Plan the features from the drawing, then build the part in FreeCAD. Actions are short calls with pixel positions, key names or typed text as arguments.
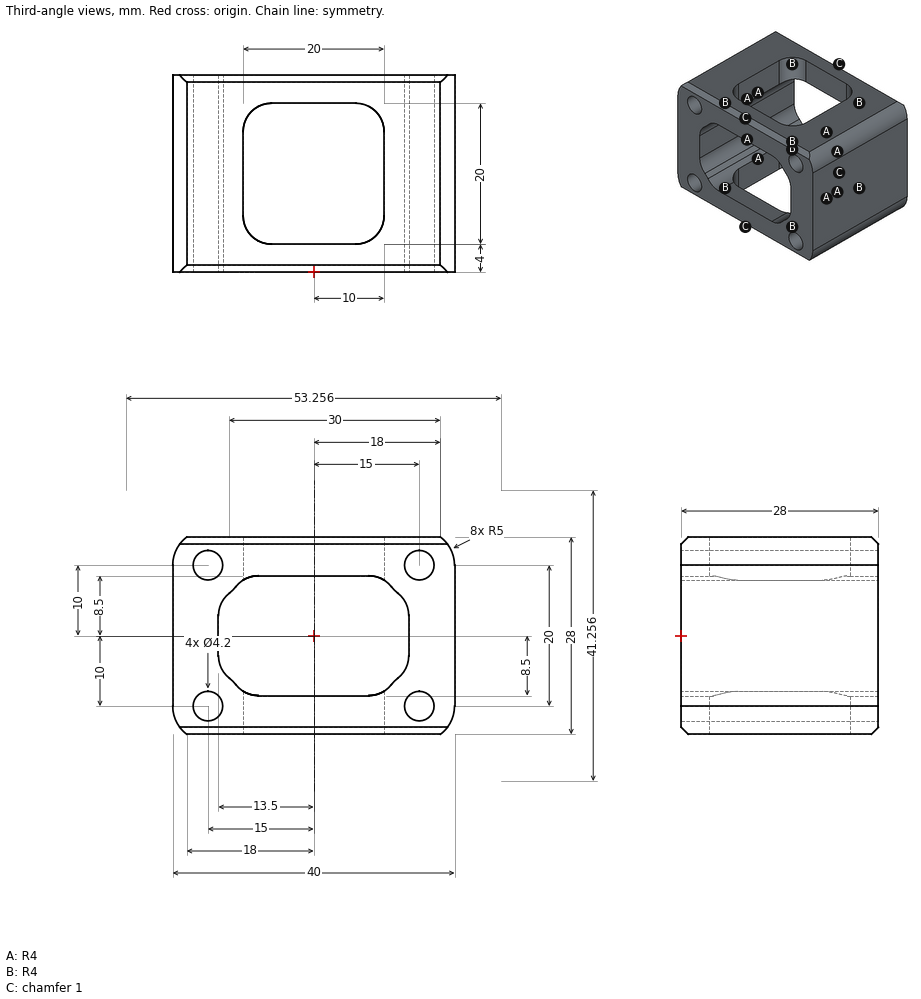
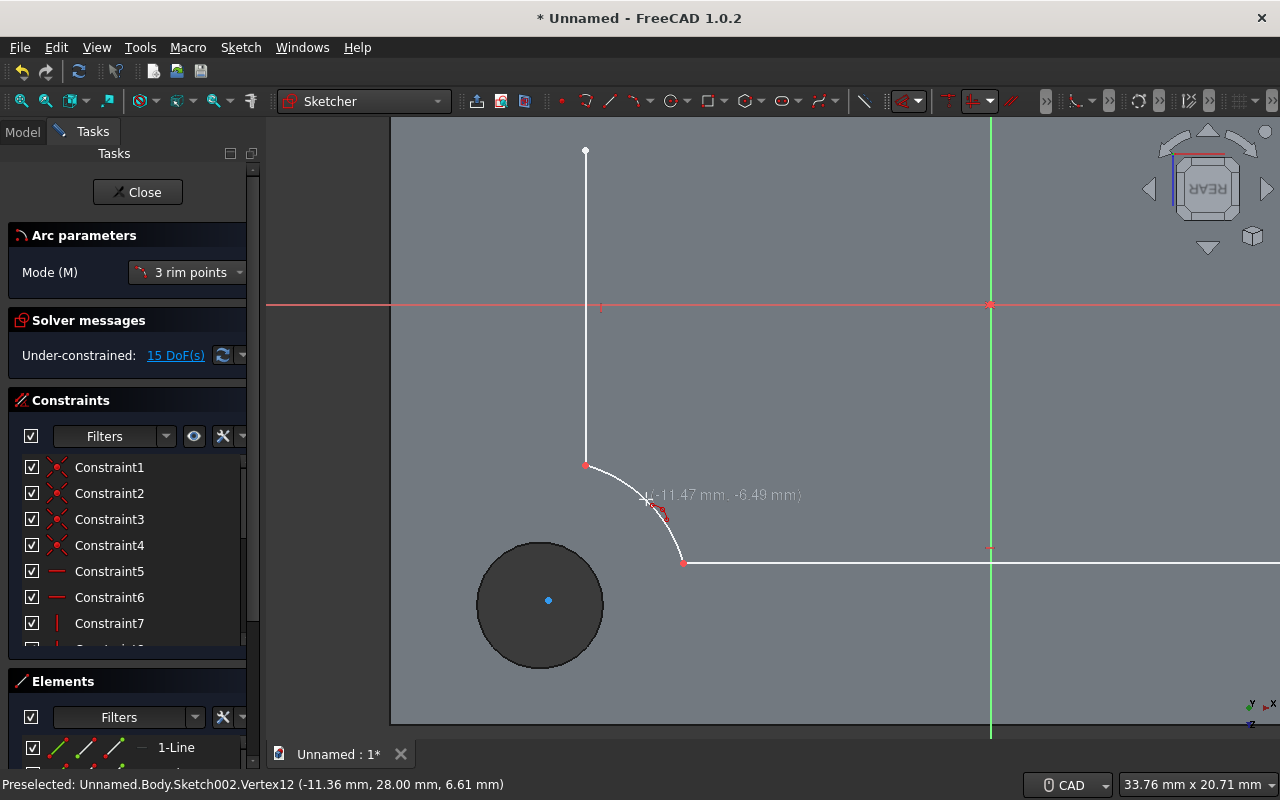
scroll(581, 481, down, 6)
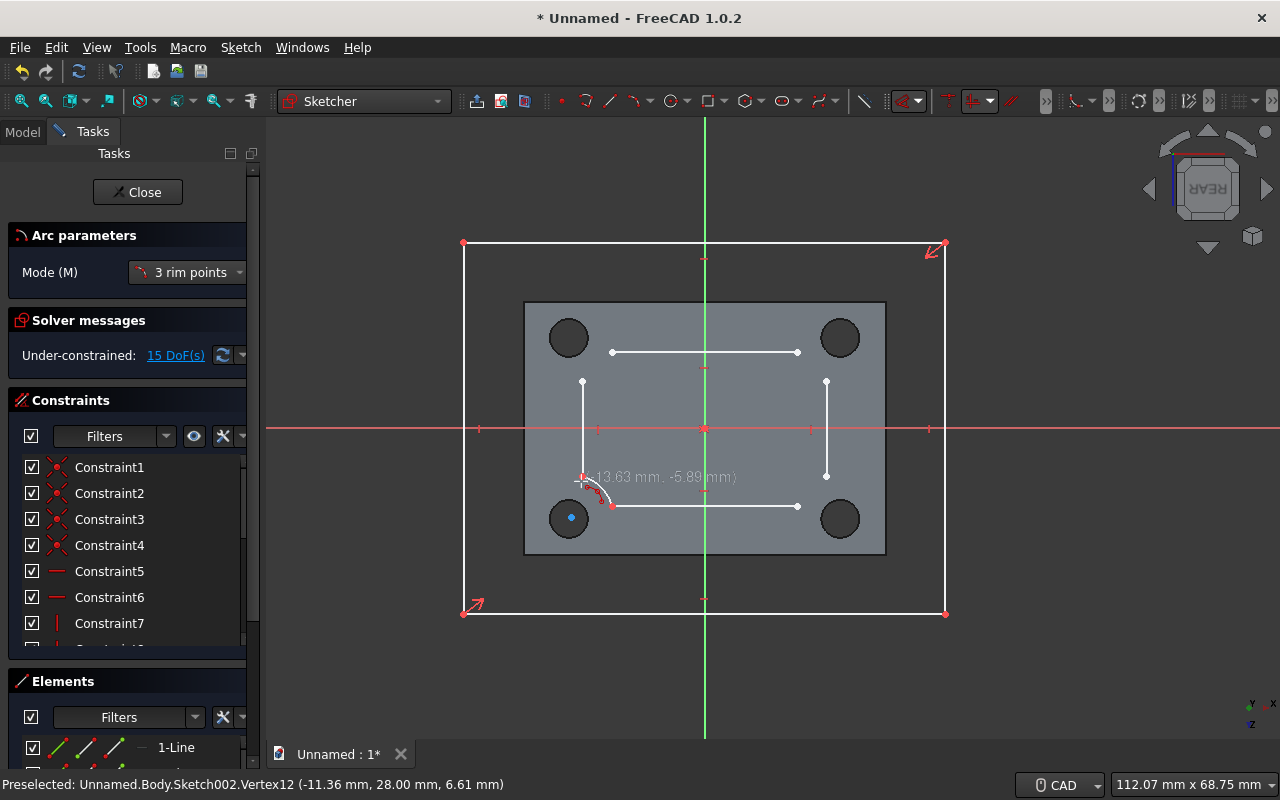
click(797, 506)
click(827, 477)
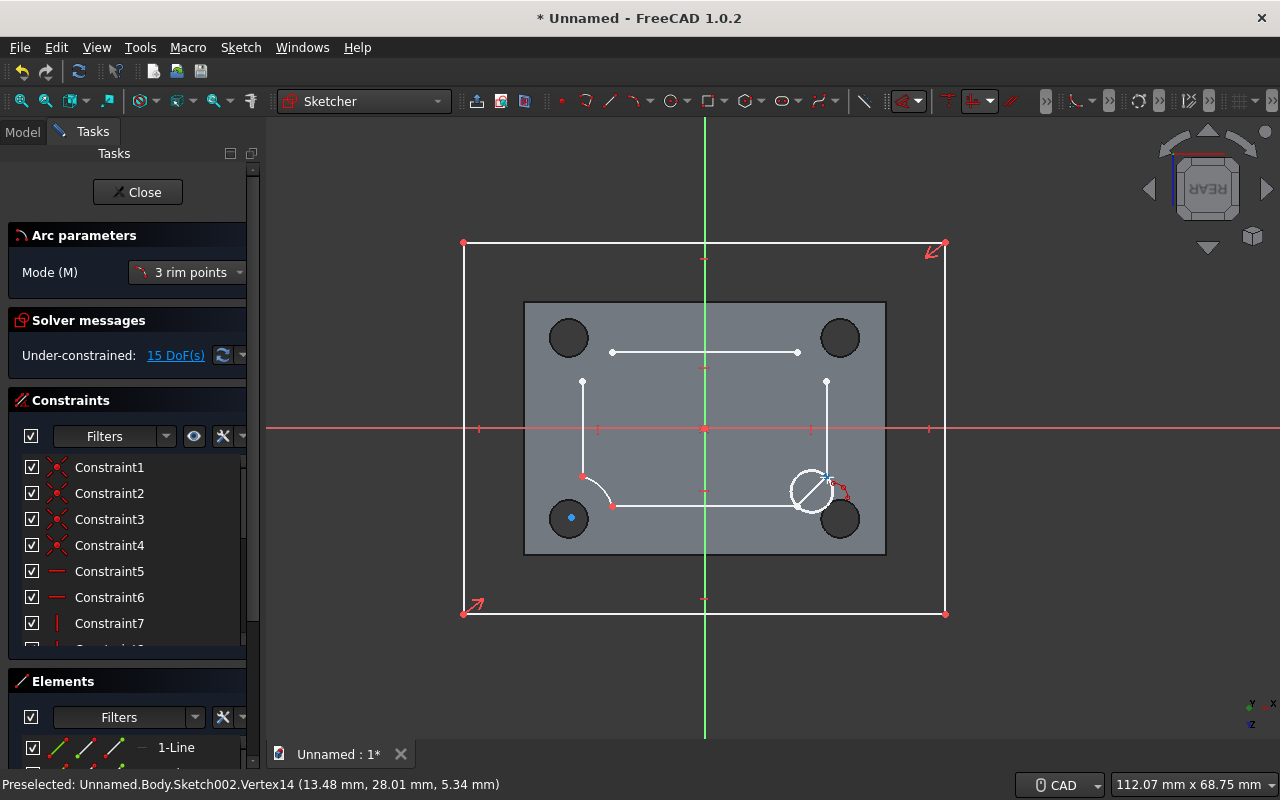
scroll(808, 487, up, 6)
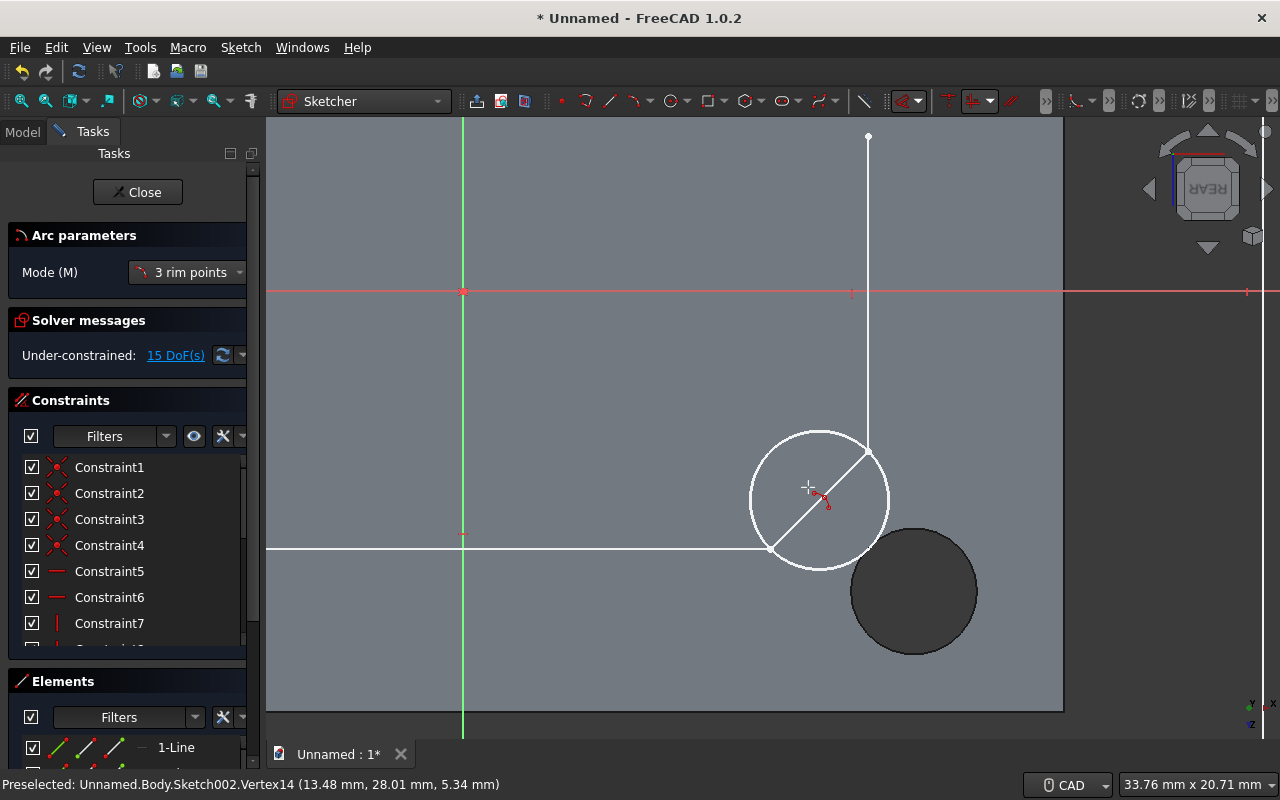
click(808, 485)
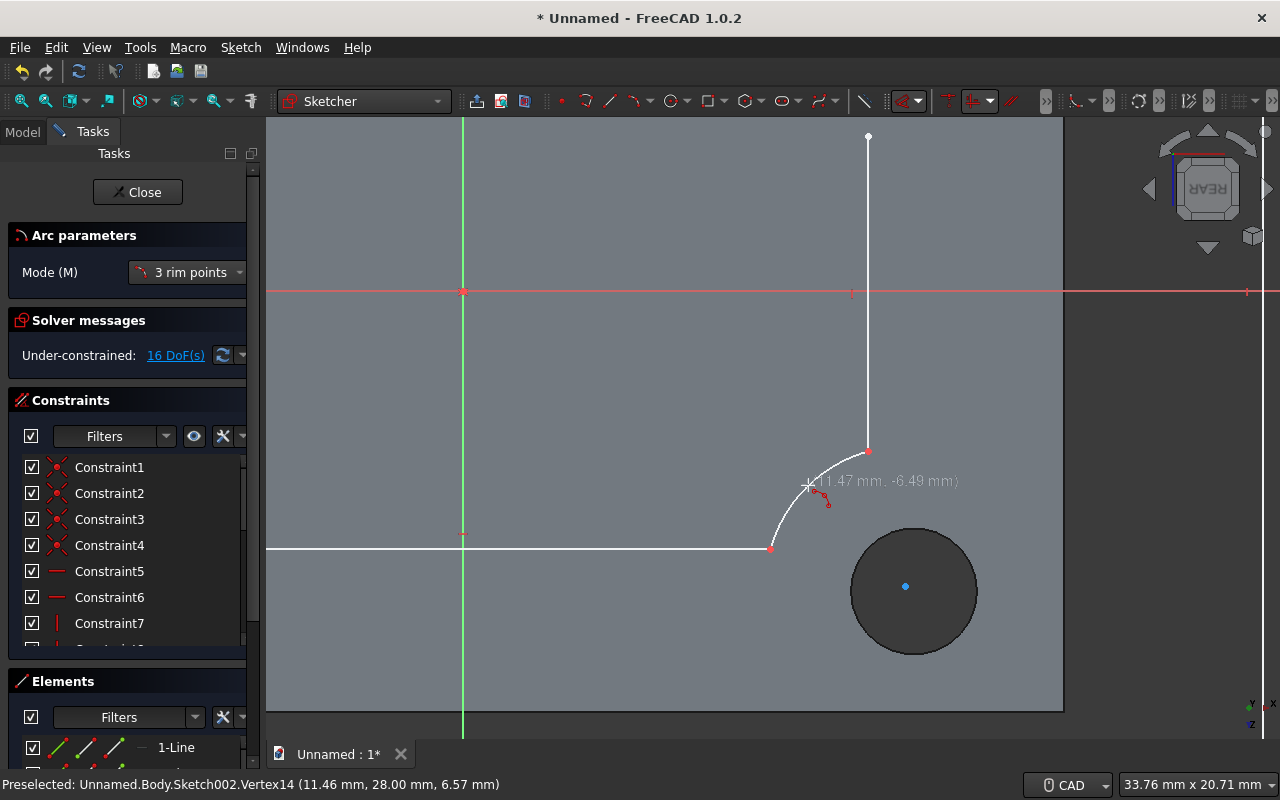
scroll(808, 487, down, 6)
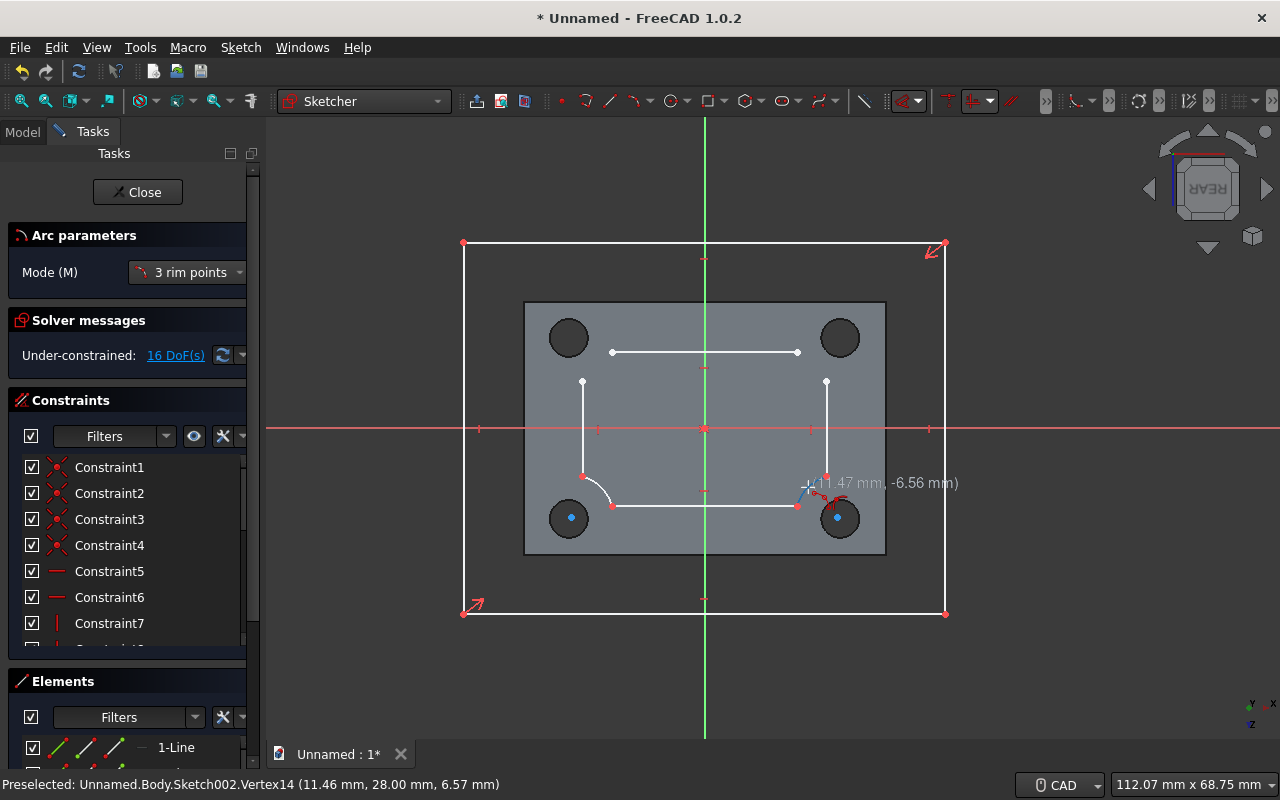
click(827, 382)
click(797, 352)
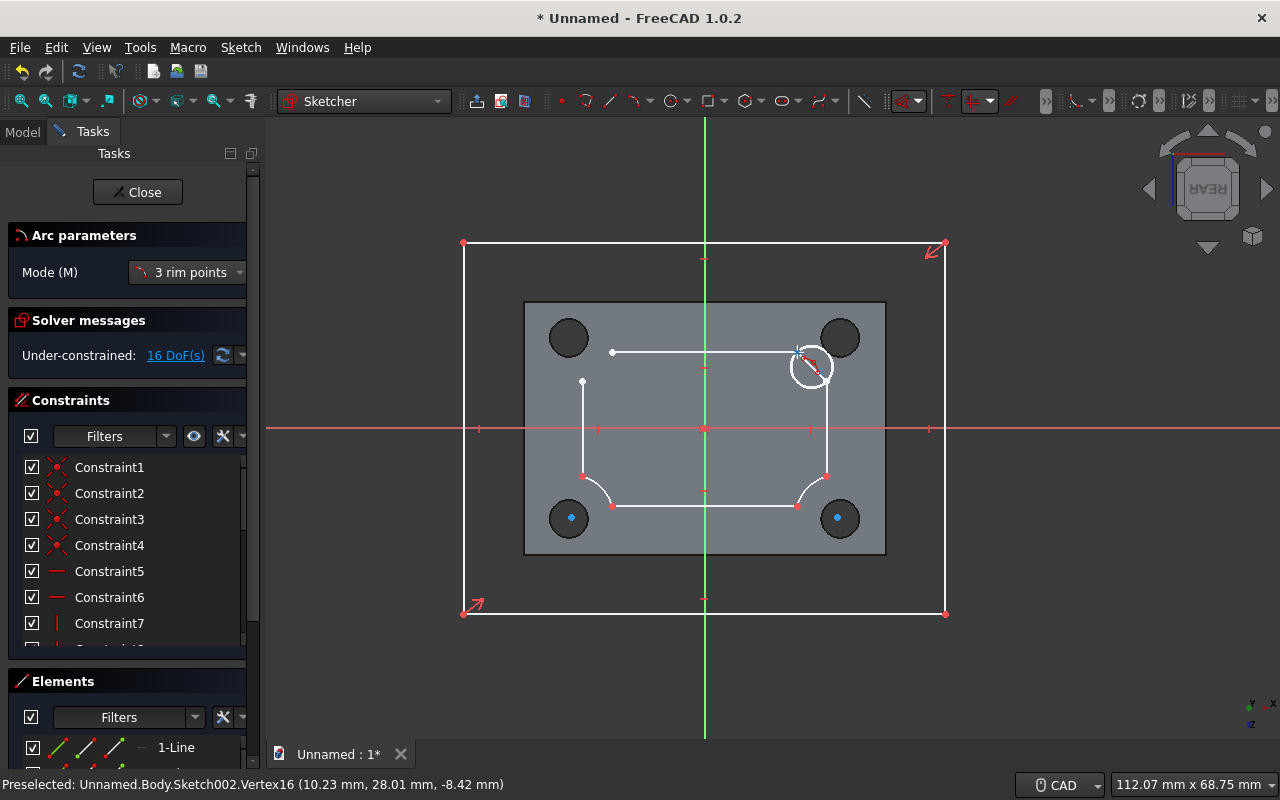
scroll(808, 370, up, 6)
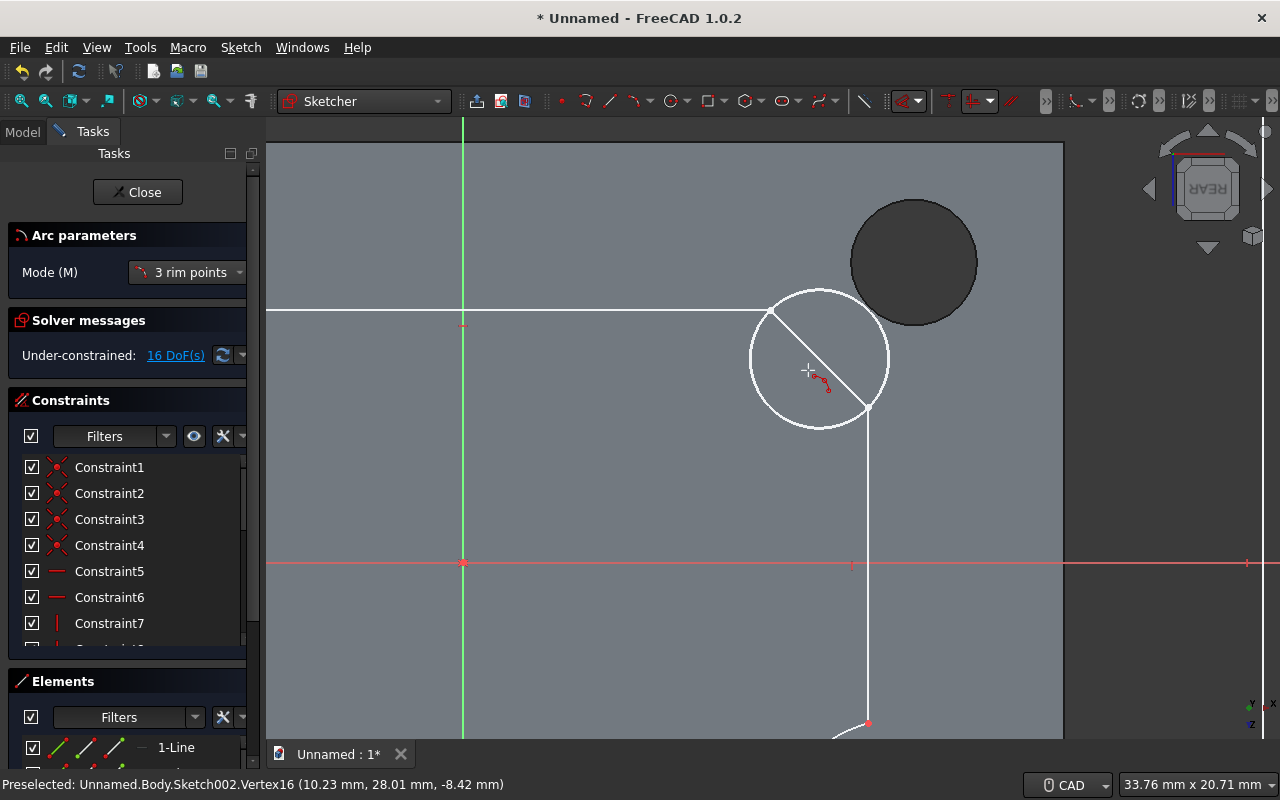
click(808, 369)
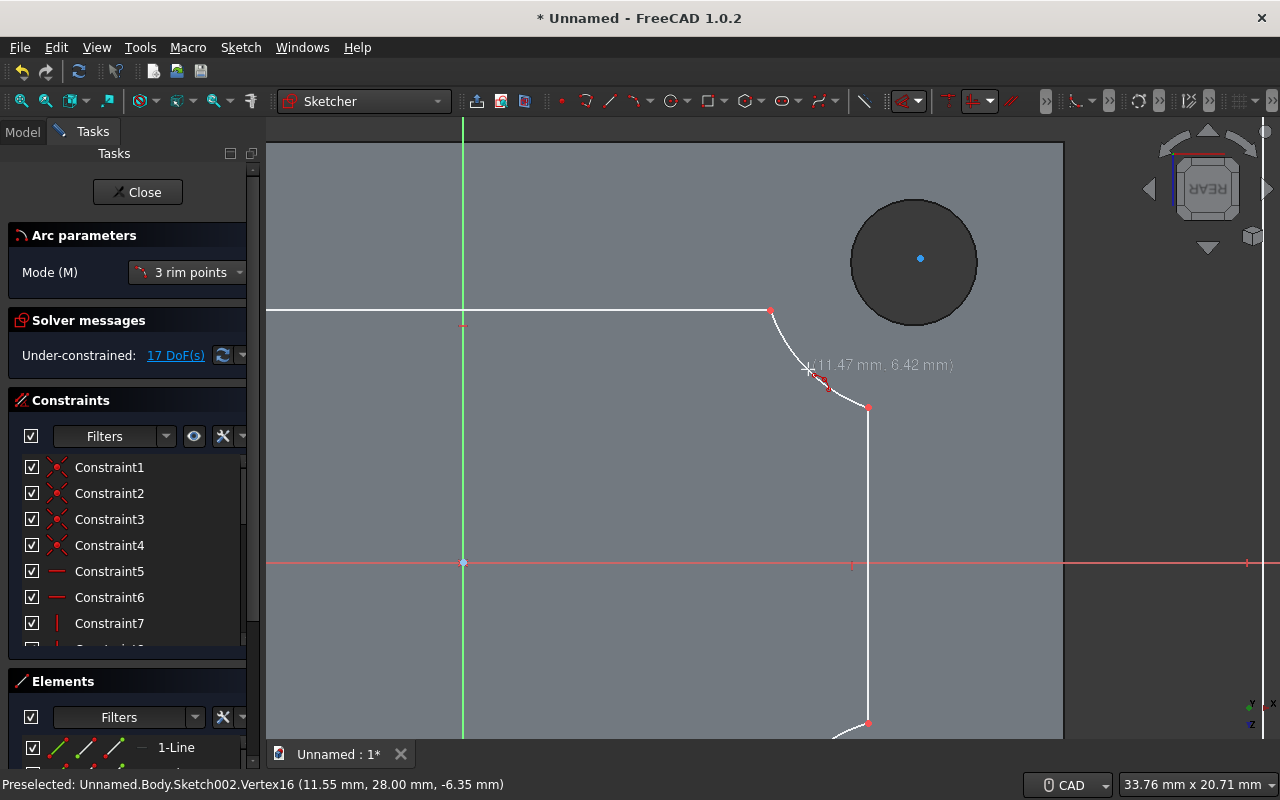
scroll(808, 370, down, 6)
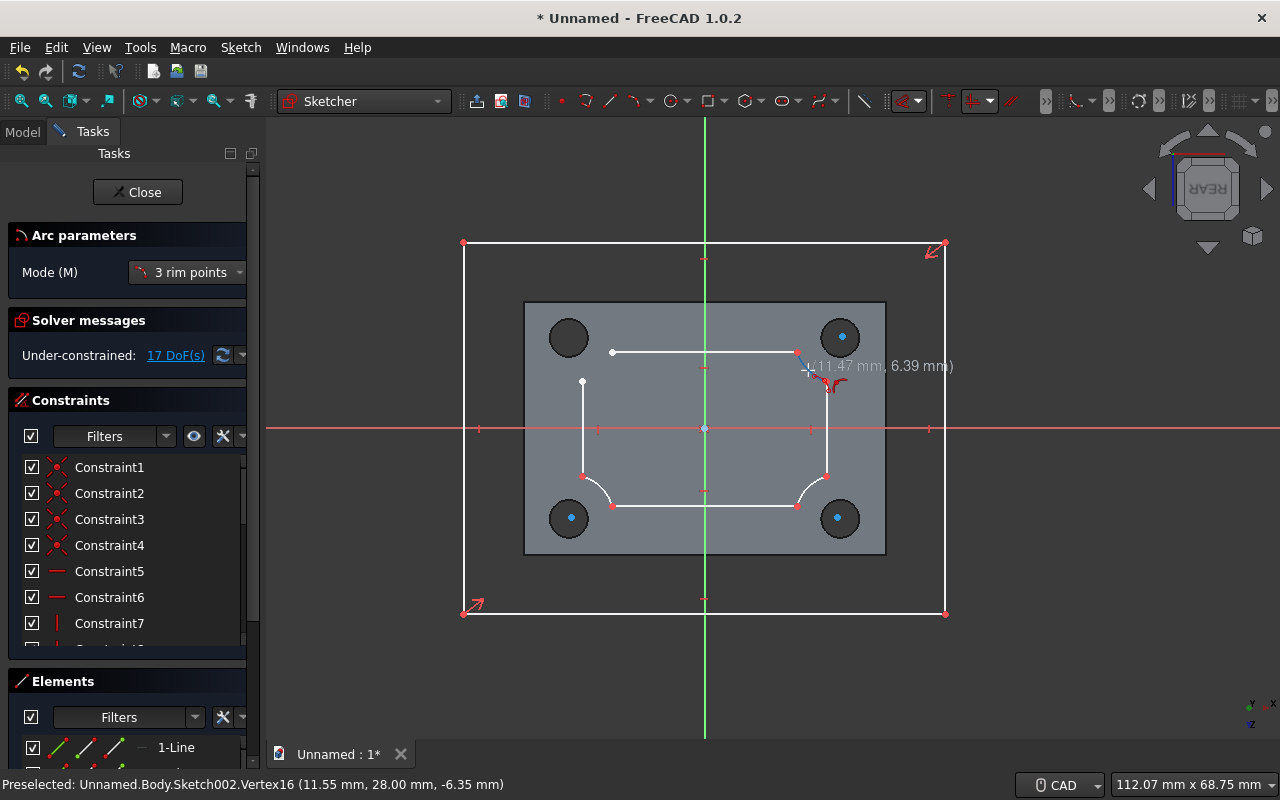
click(612, 352)
click(583, 382)